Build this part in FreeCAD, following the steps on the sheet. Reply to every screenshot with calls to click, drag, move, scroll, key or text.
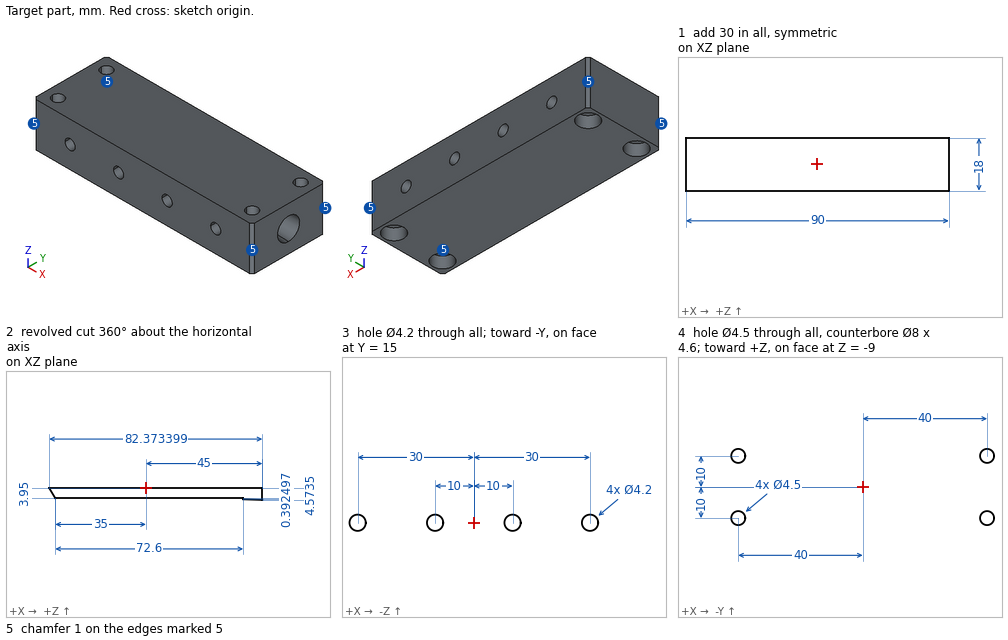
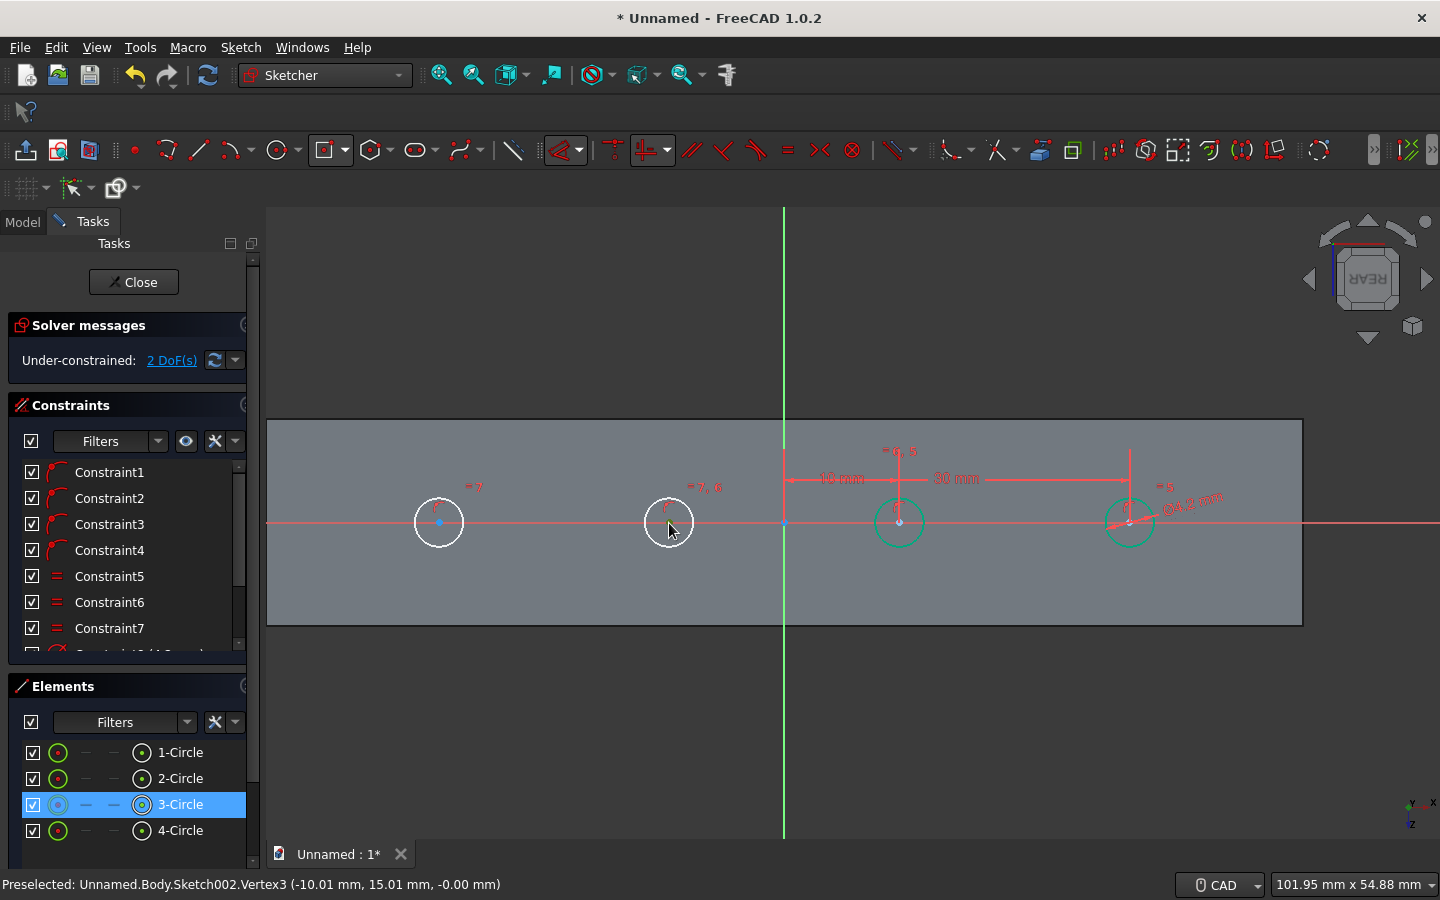
click(582, 150)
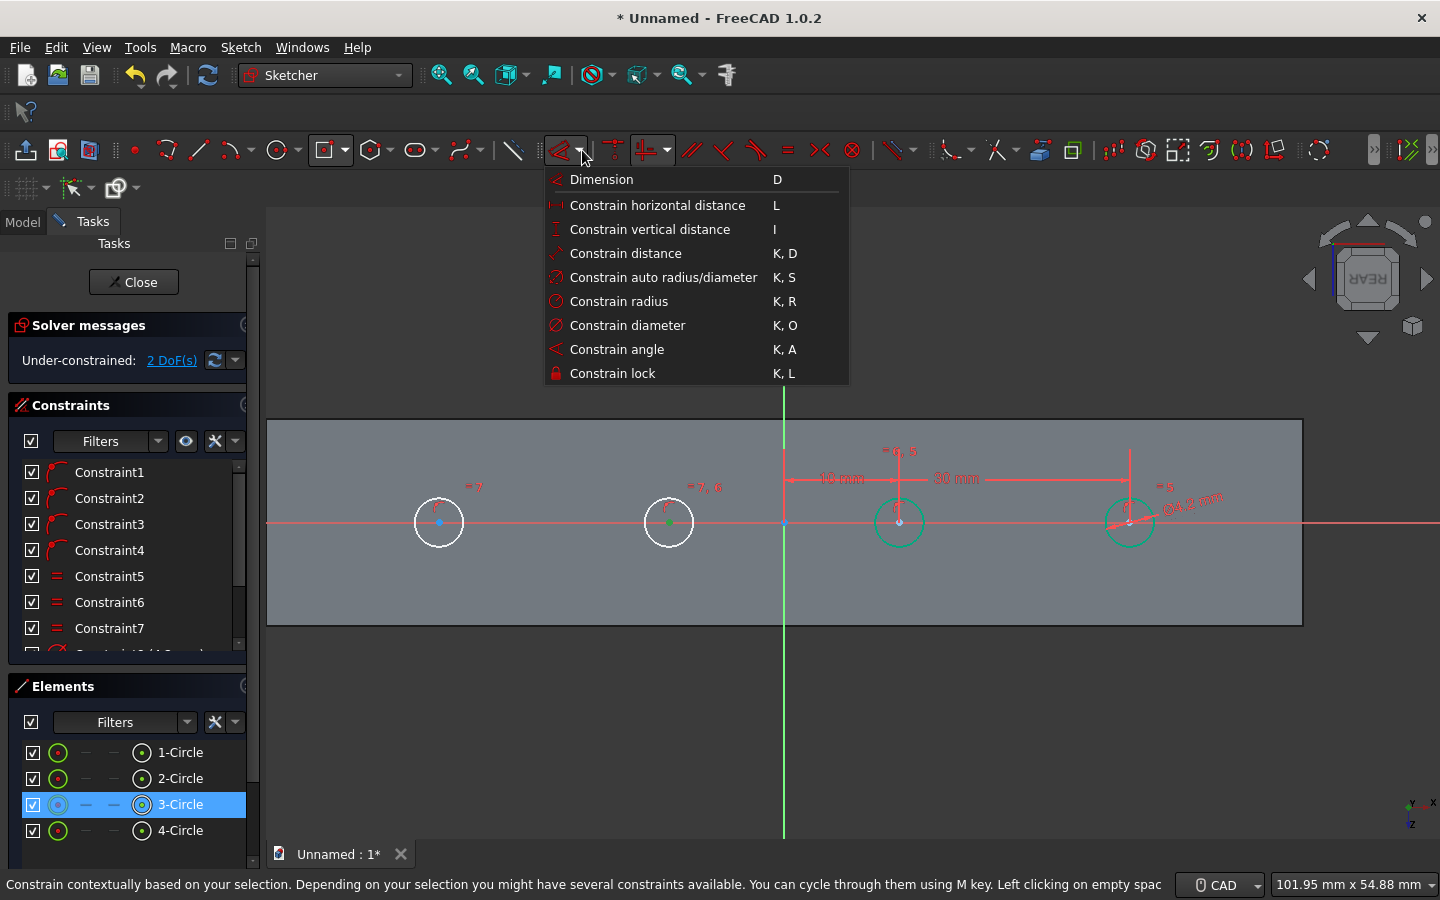
click(697, 205)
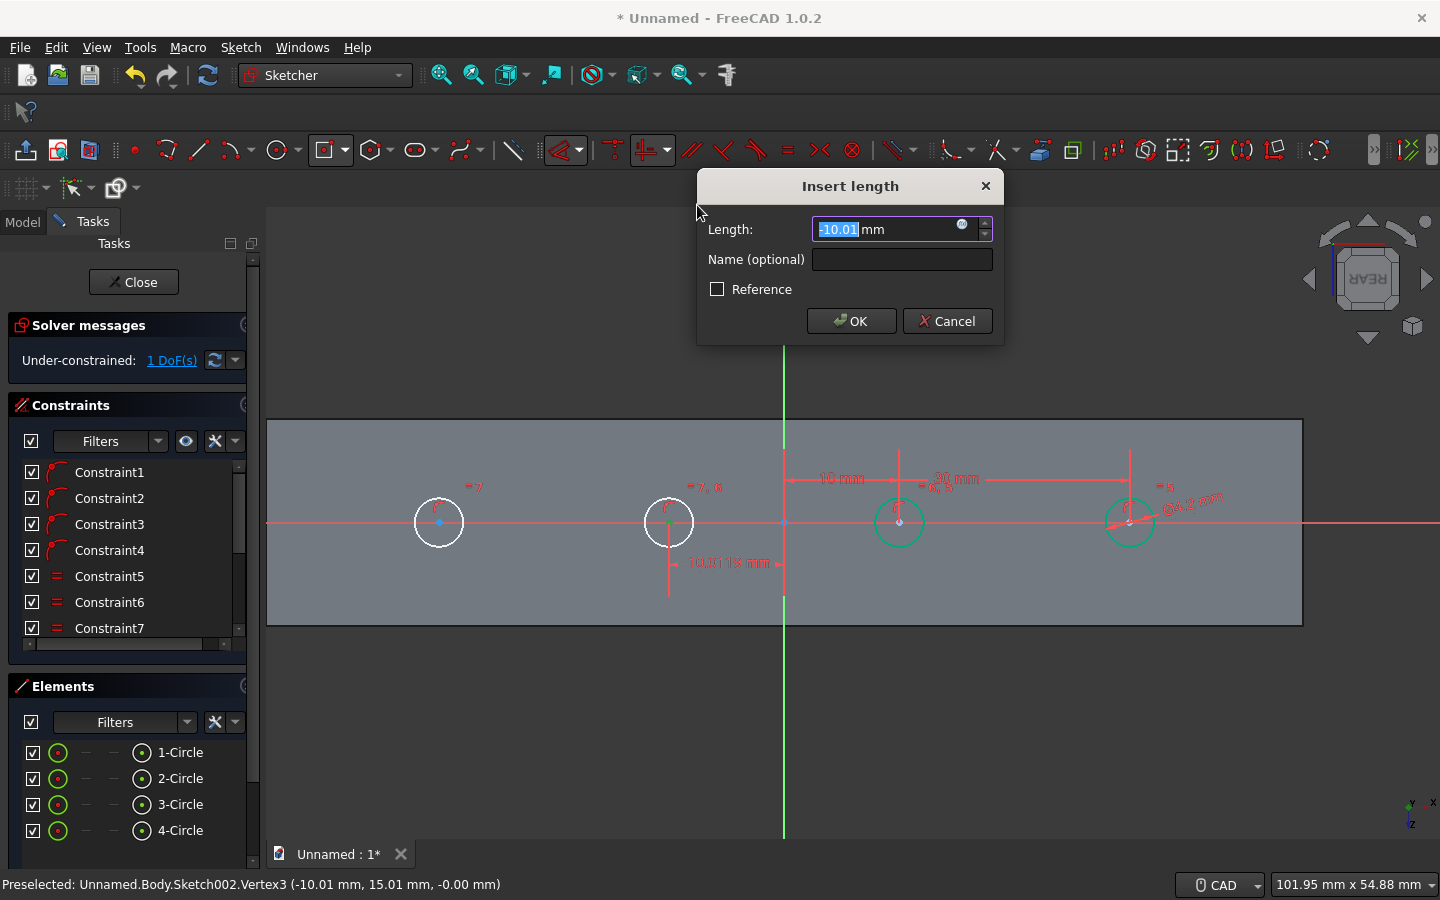
text(-10)
key(Return)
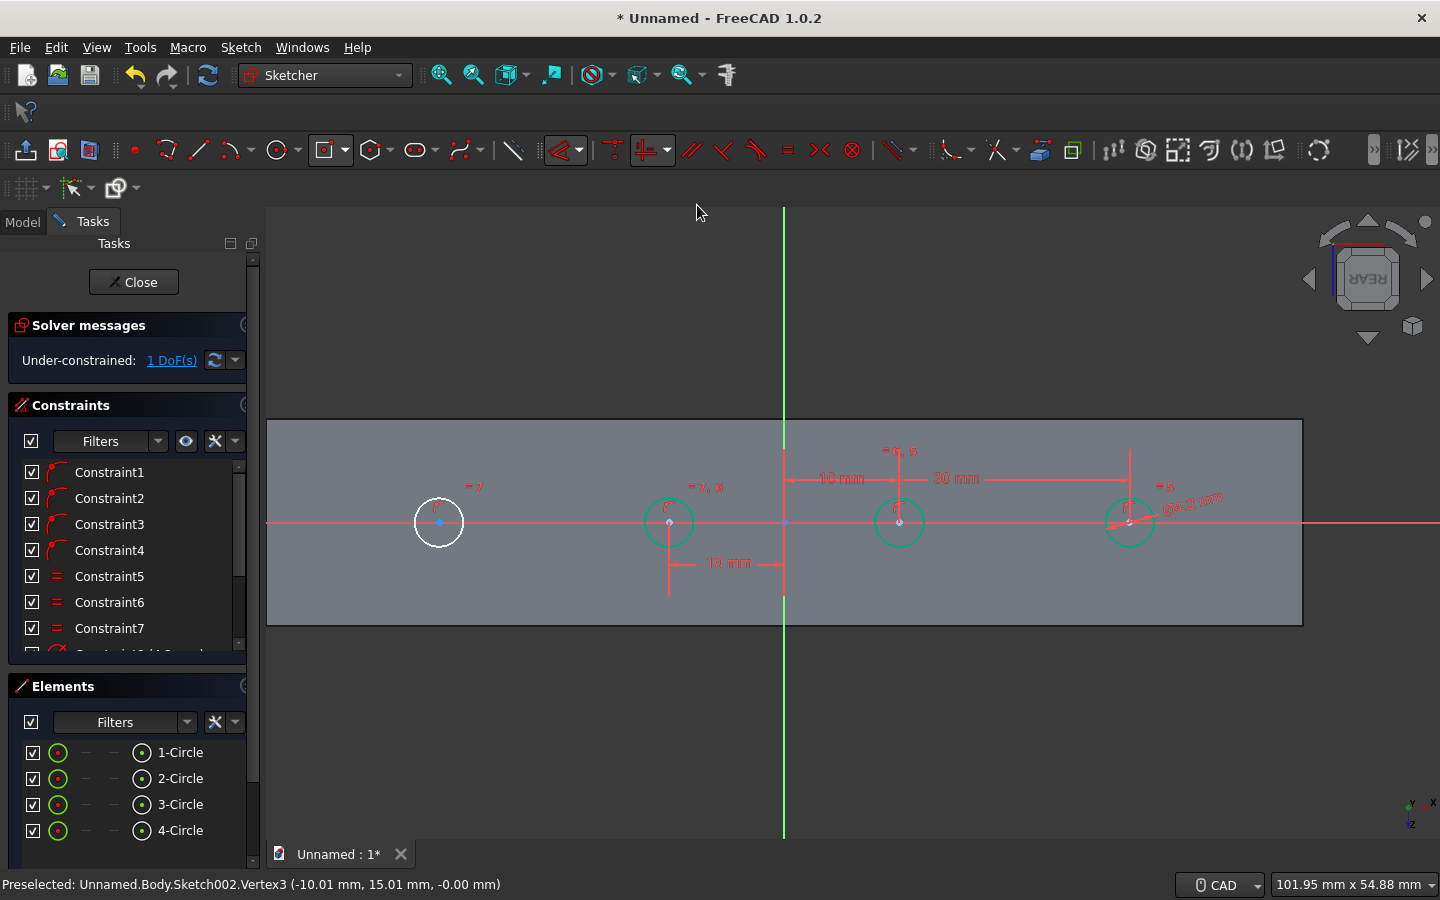
click(439, 523)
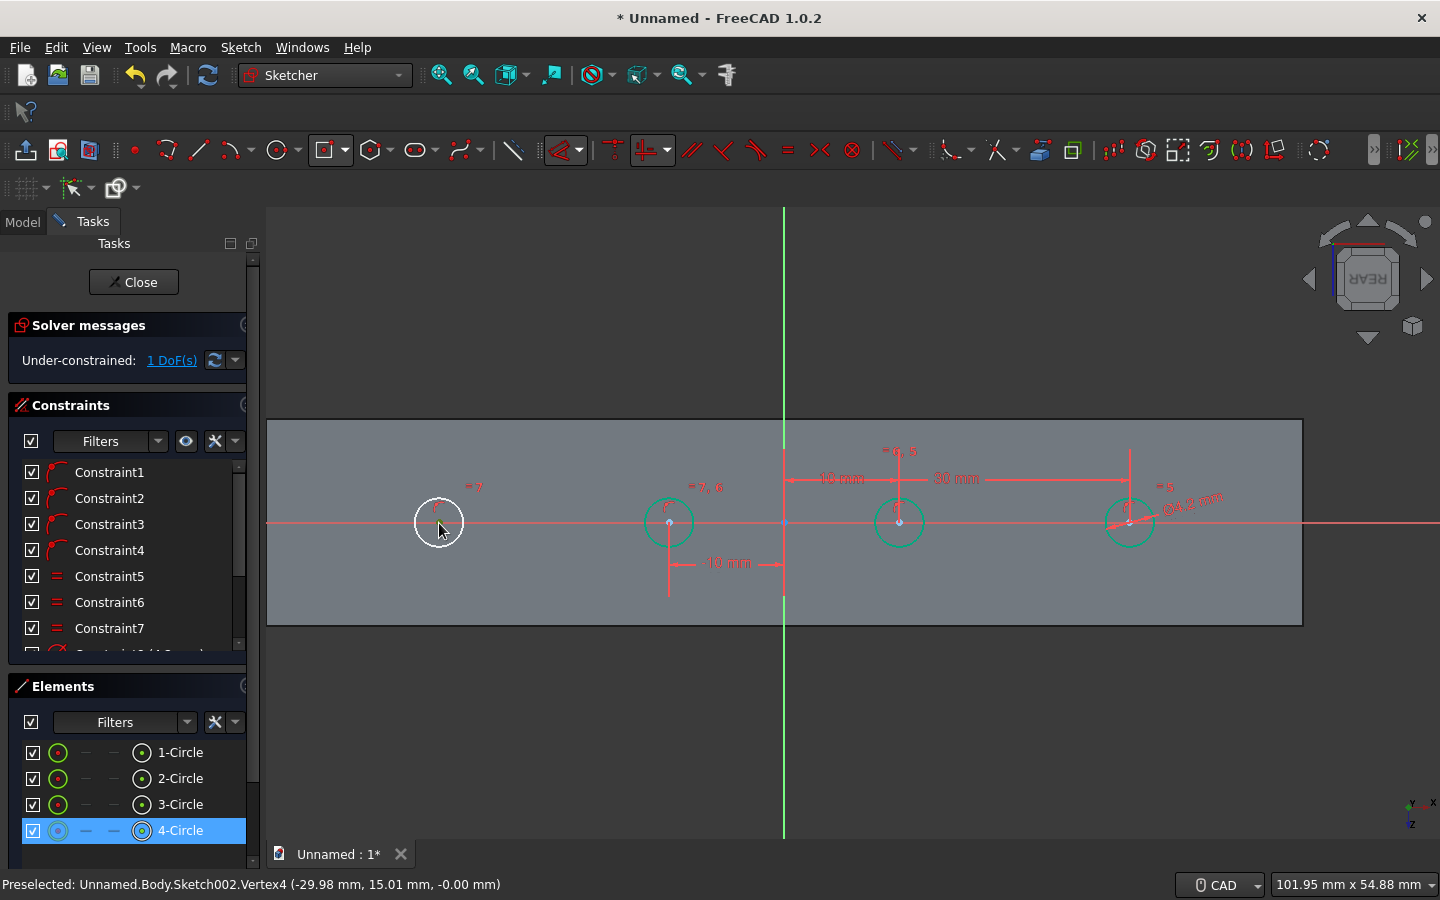
key(l)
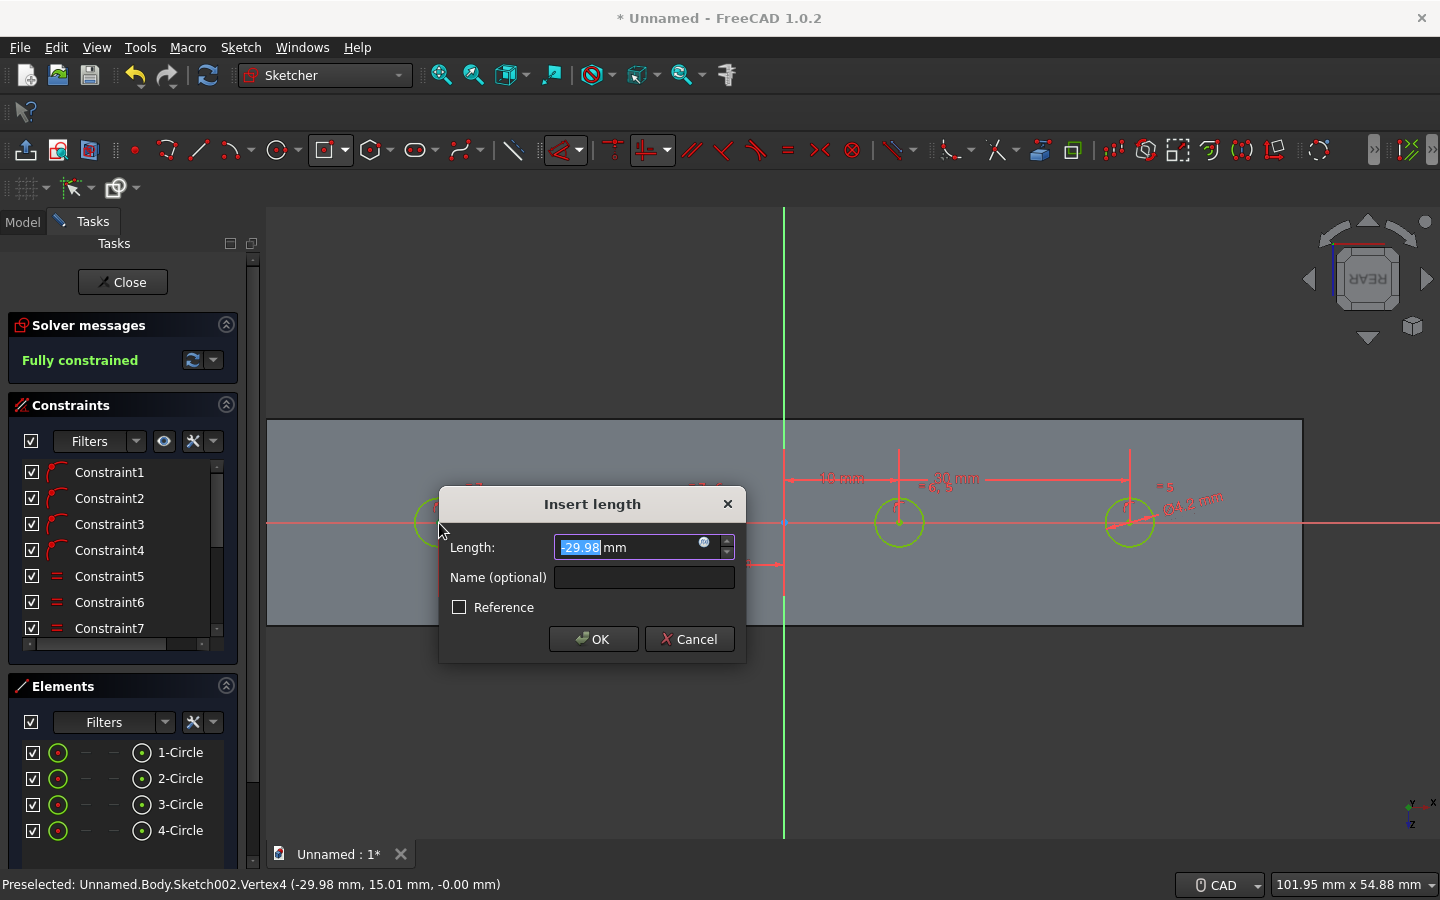
text(-30)
key(Return)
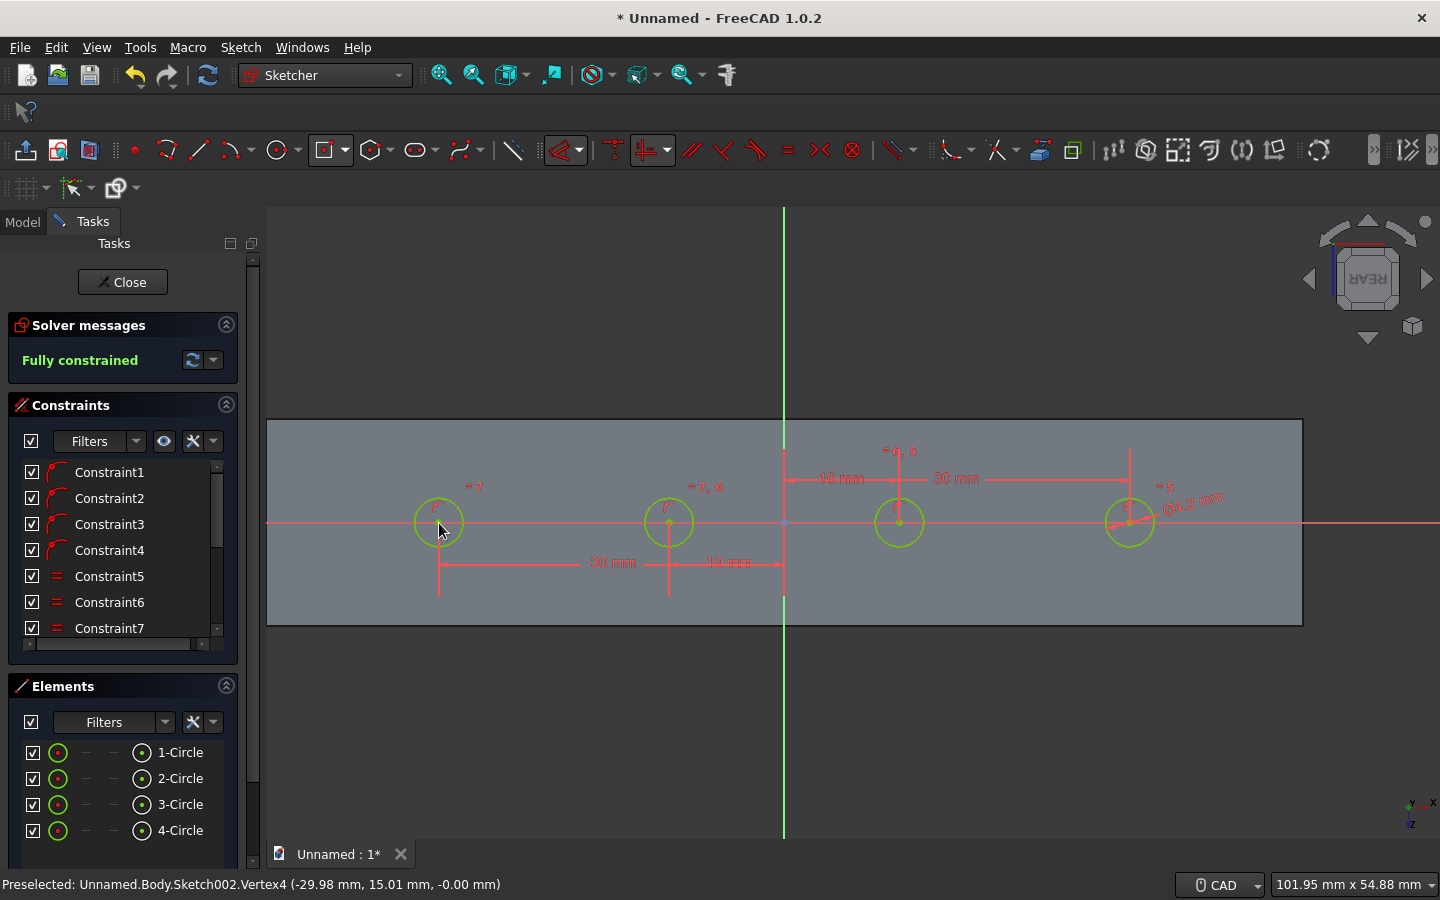
click(123, 282)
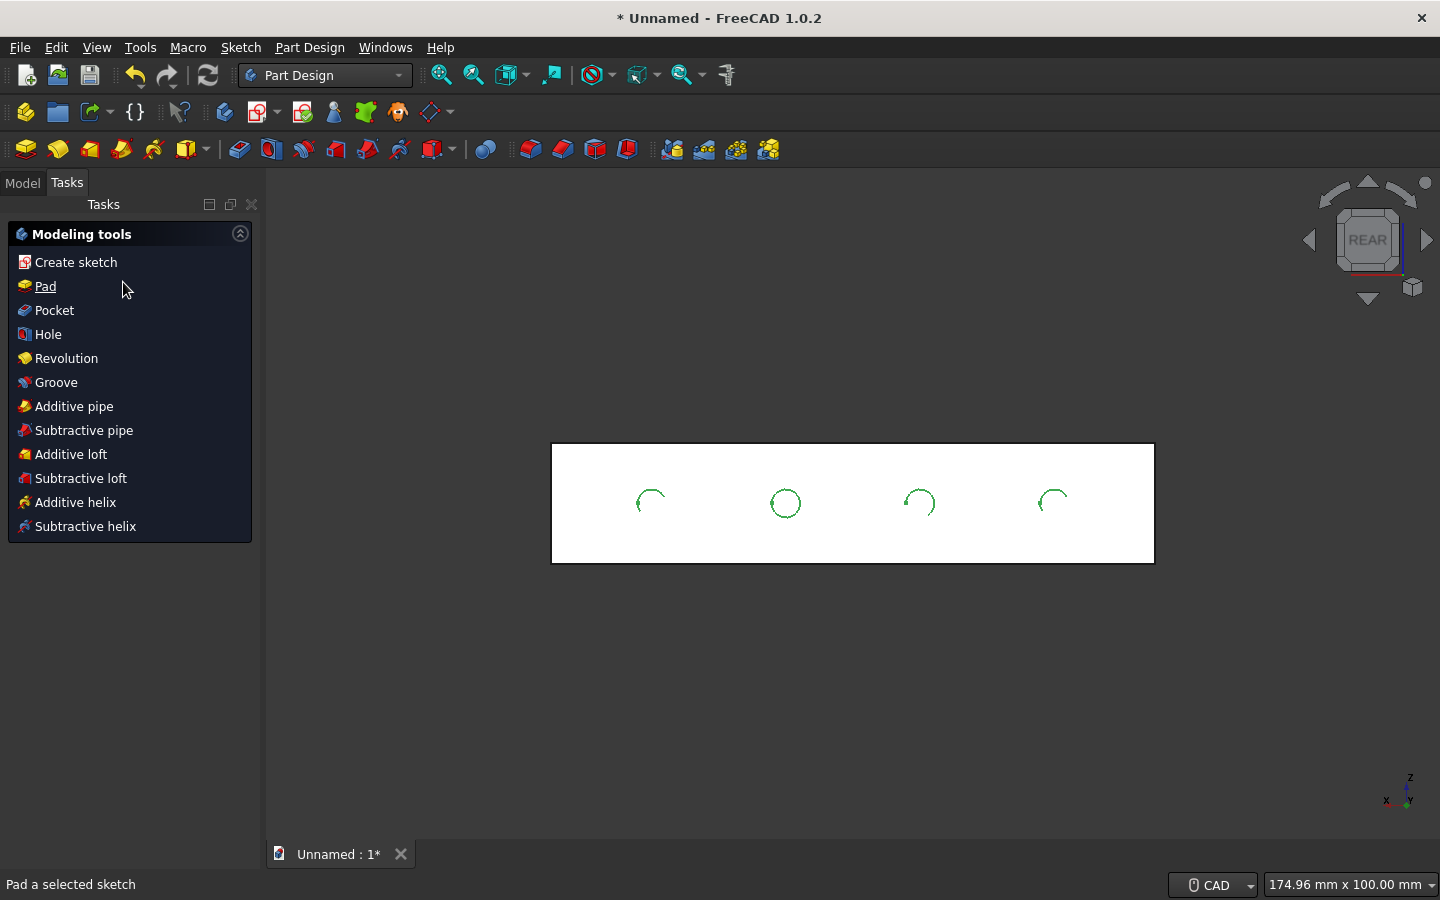
click(272, 150)